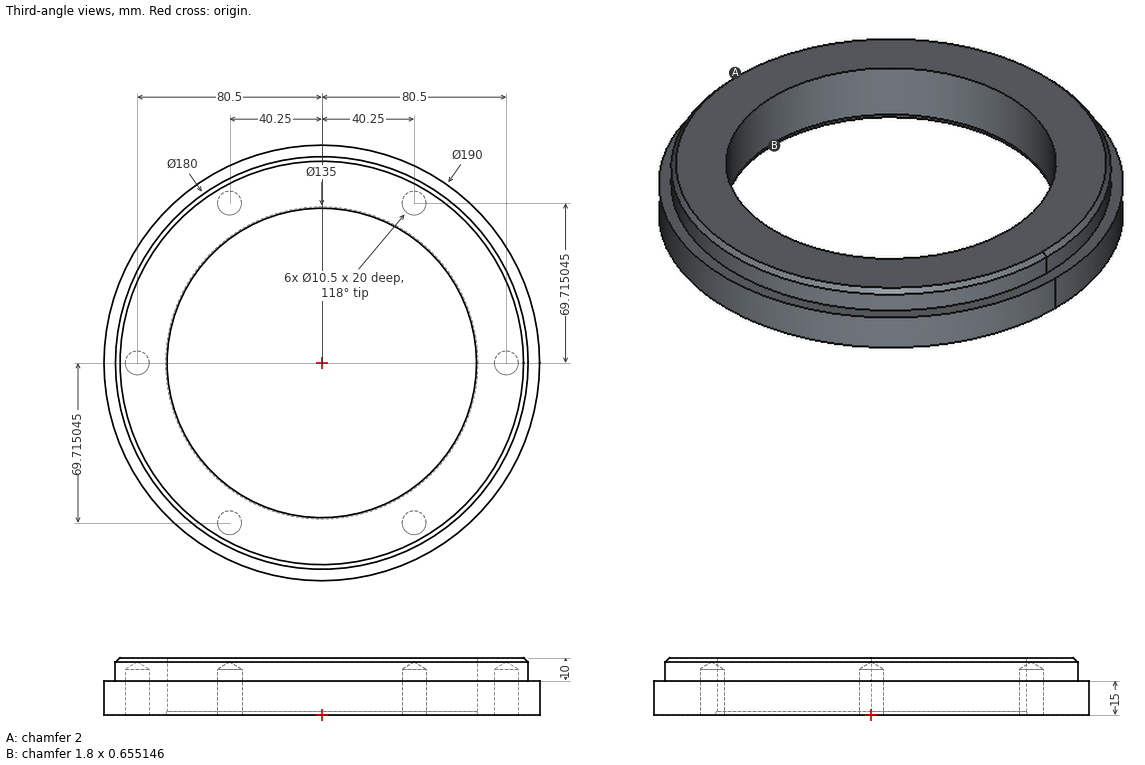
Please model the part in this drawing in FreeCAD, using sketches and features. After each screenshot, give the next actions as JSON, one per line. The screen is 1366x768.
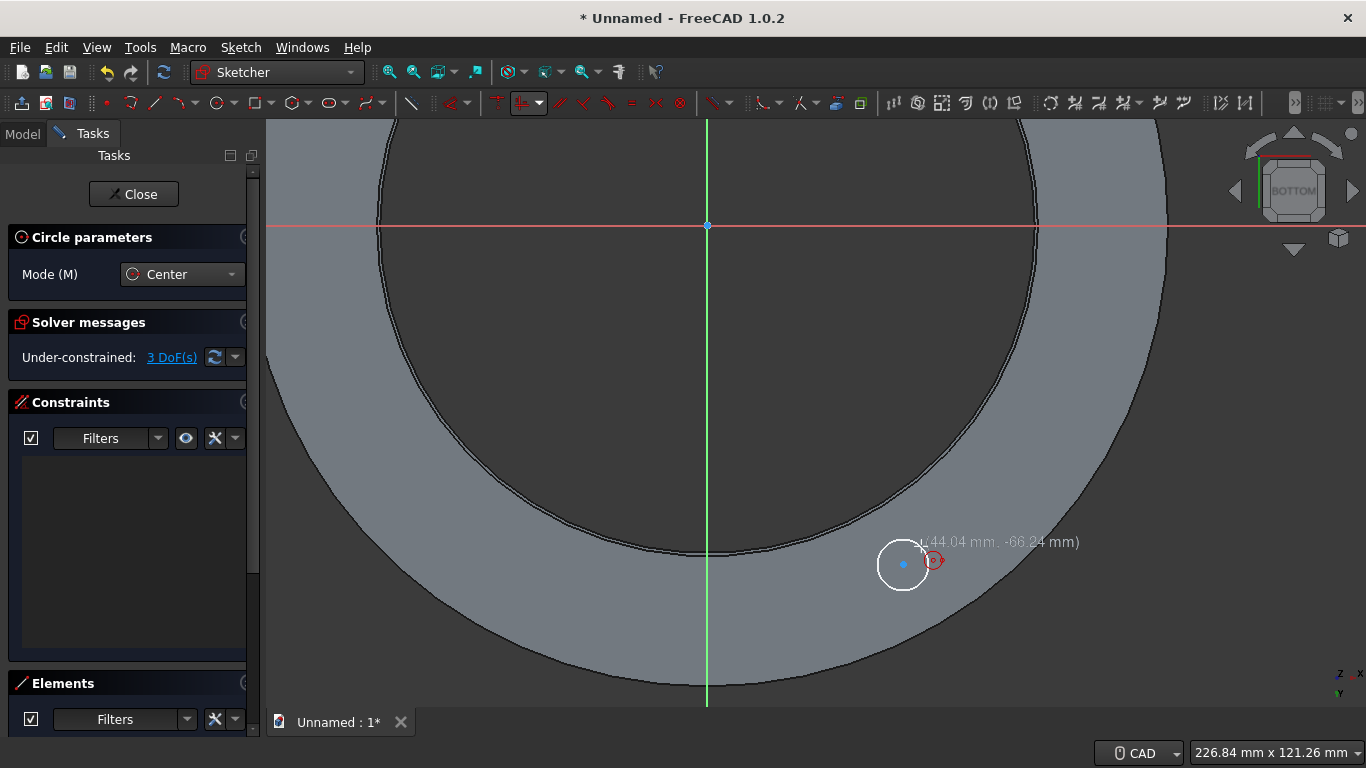
{"action": "left_click", "coordinate": [512, 564]}
{"action": "left_click", "coordinate": [530, 546]}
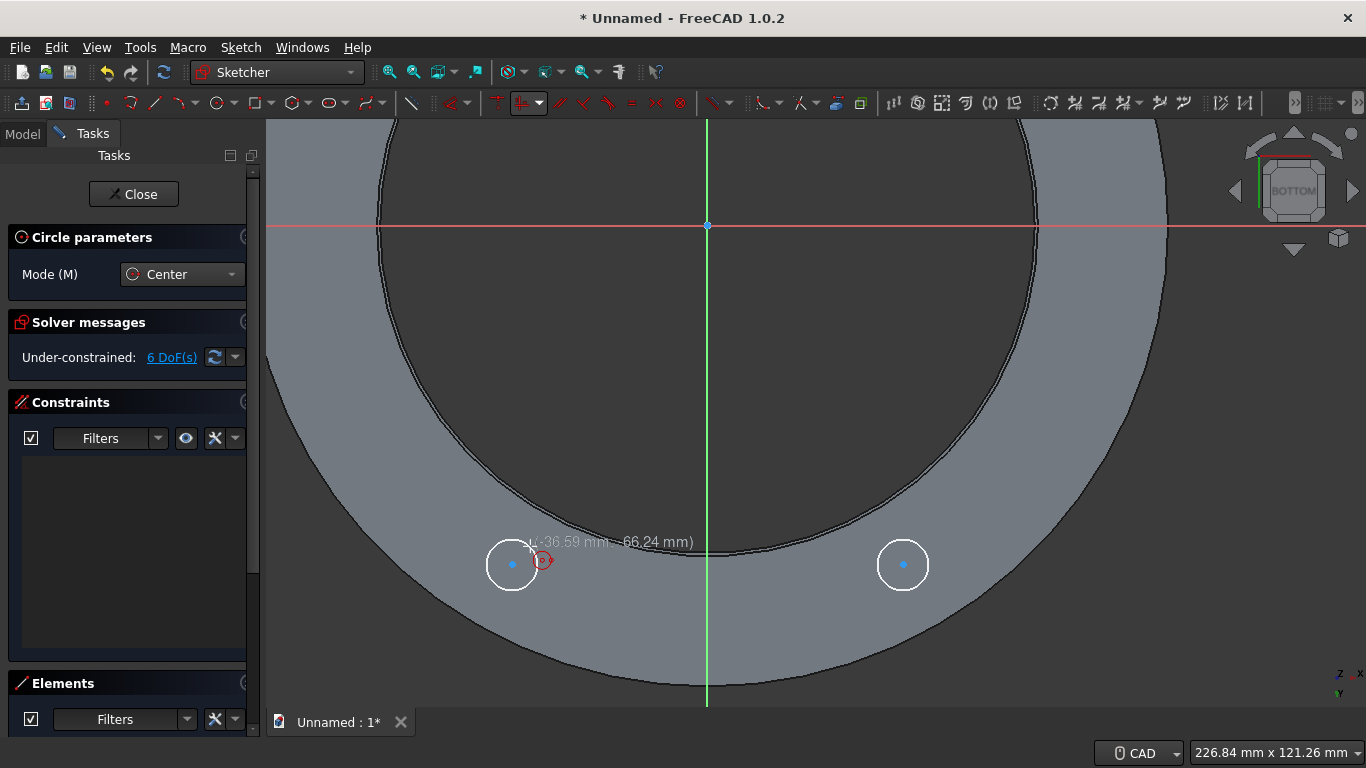
{"action": "left_click", "coordinate": [317, 226]}
{"action": "left_click", "coordinate": [335, 208]}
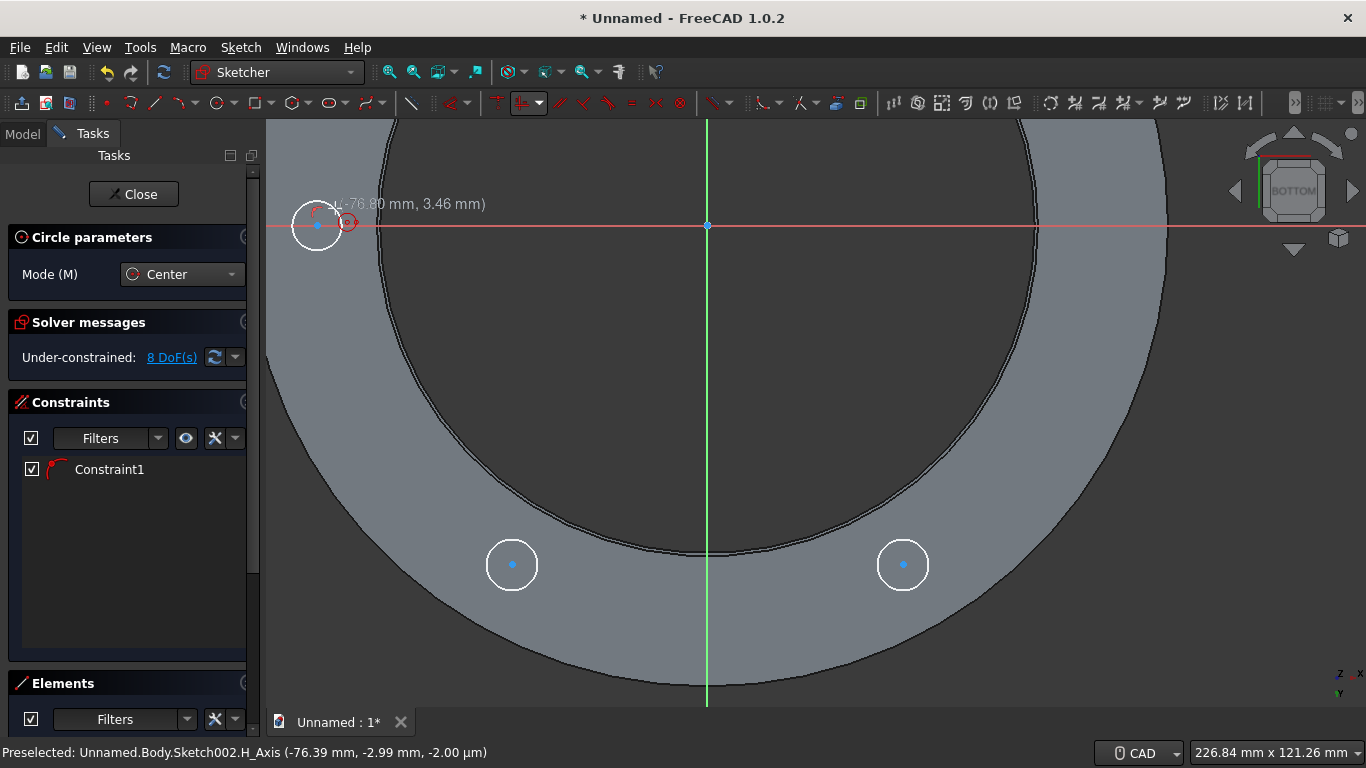
{"action": "scroll", "coordinate": [796, 641], "scroll_direction": "down", "scroll_amount": 3}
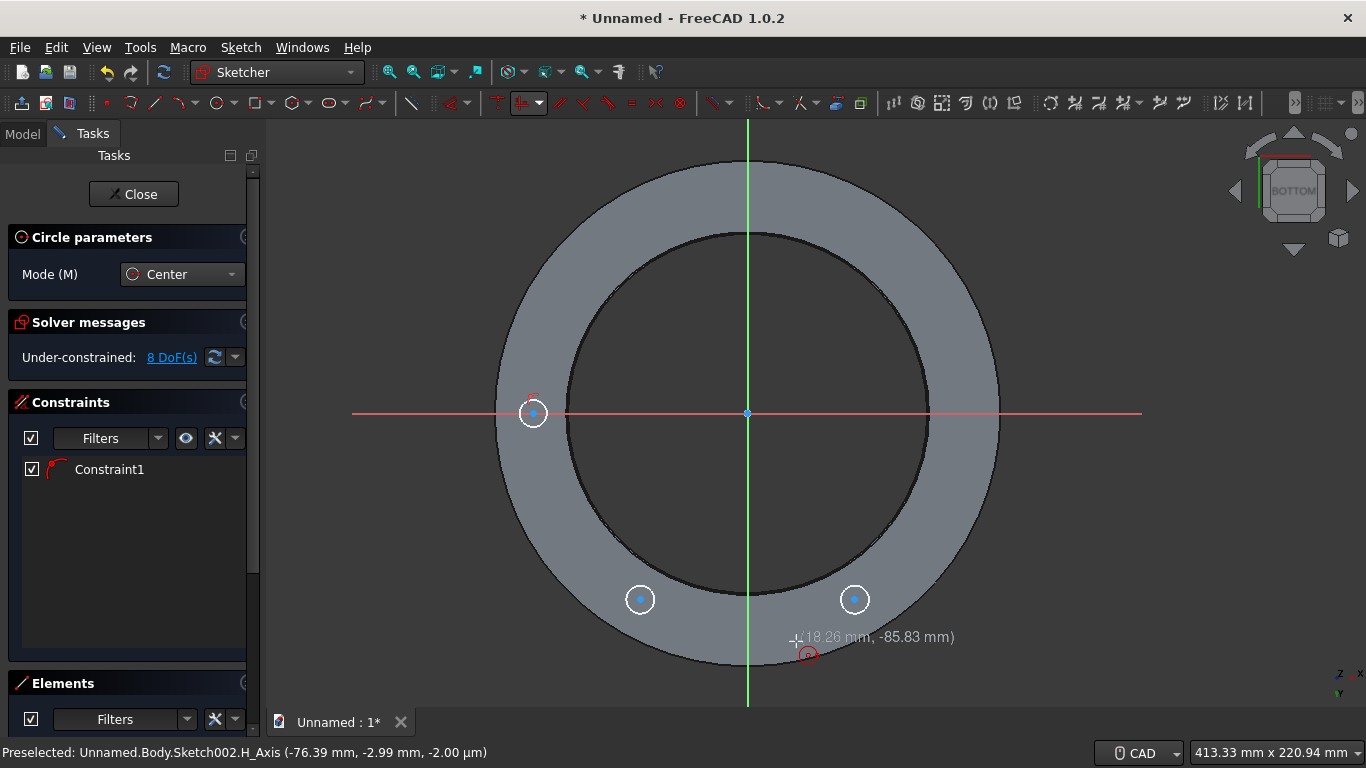
{"action": "scroll", "coordinate": [640, 228], "scroll_direction": "up", "scroll_amount": 3}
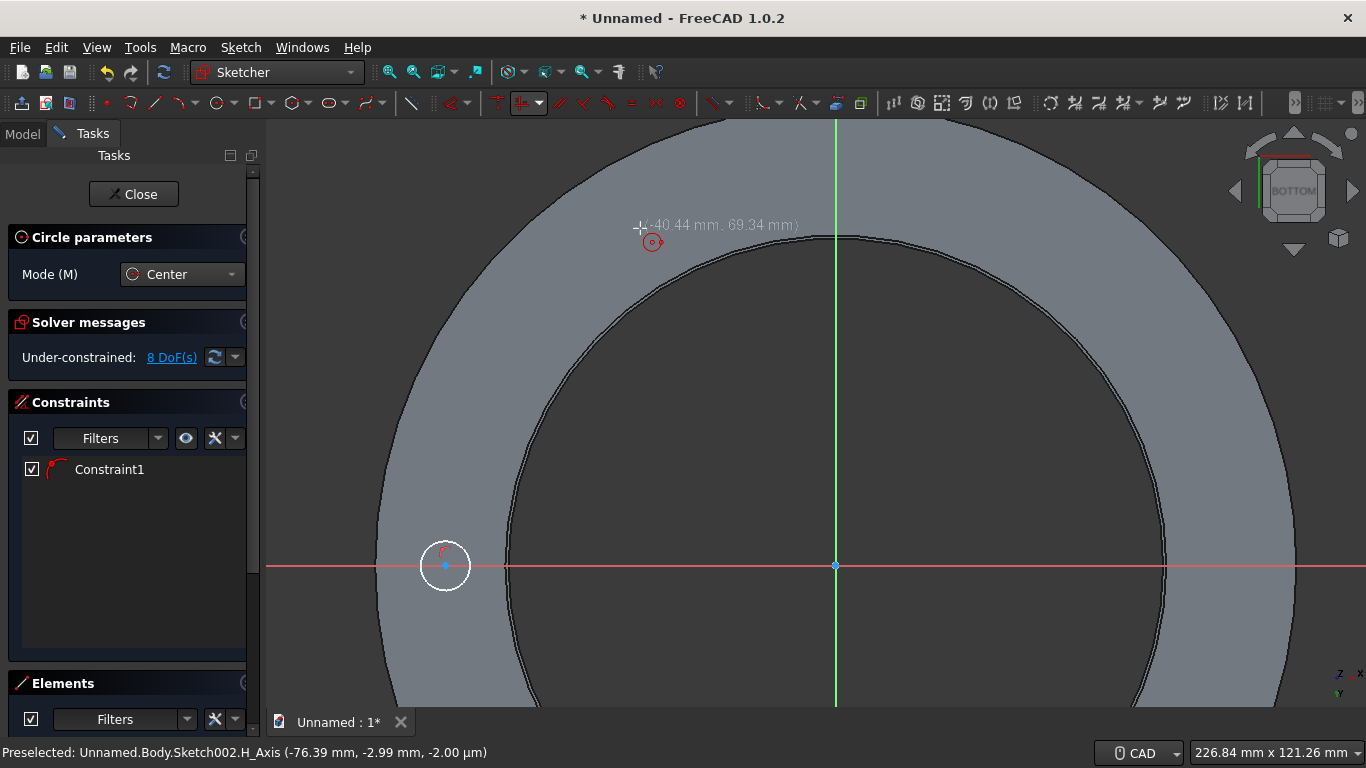
{"action": "left_click", "coordinate": [641, 228]}
{"action": "left_click", "coordinate": [659, 210]}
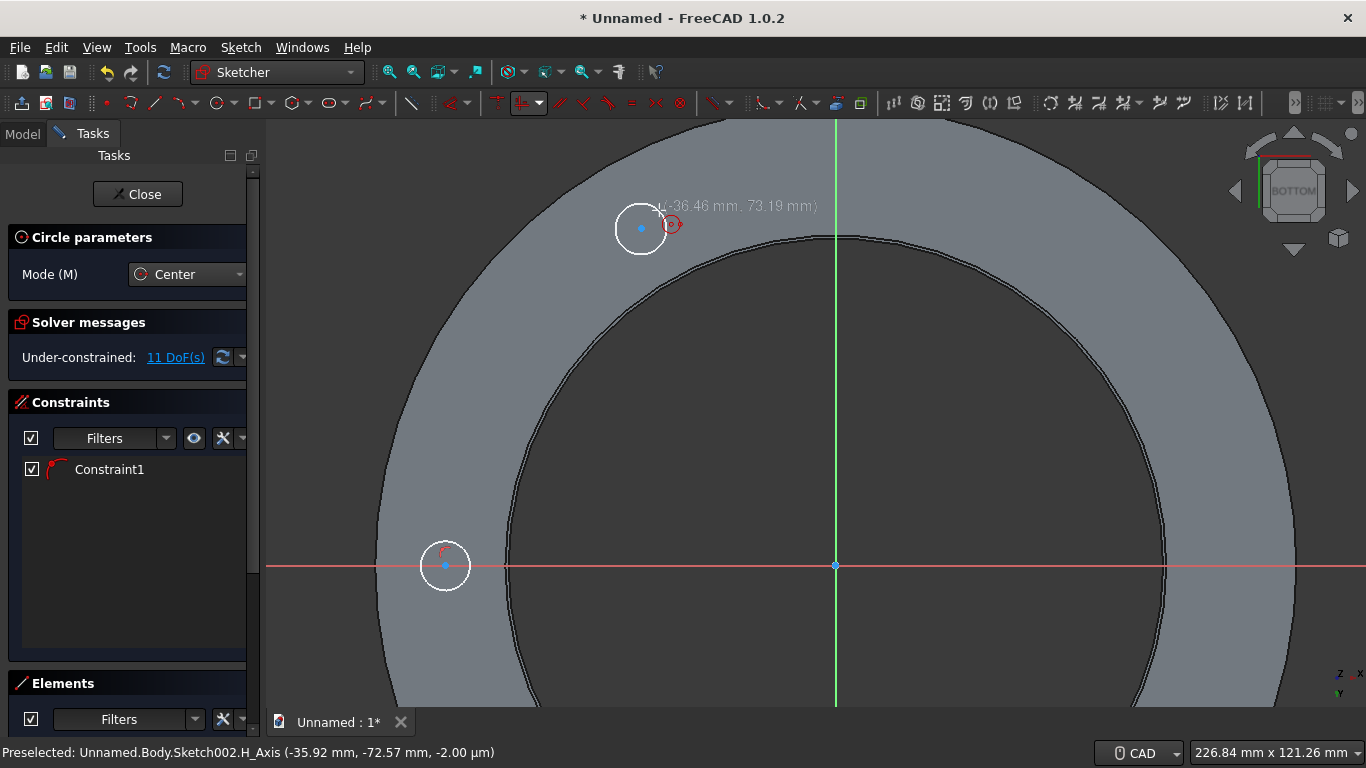
{"action": "scroll", "coordinate": [640, 227], "scroll_direction": "down", "scroll_amount": 3}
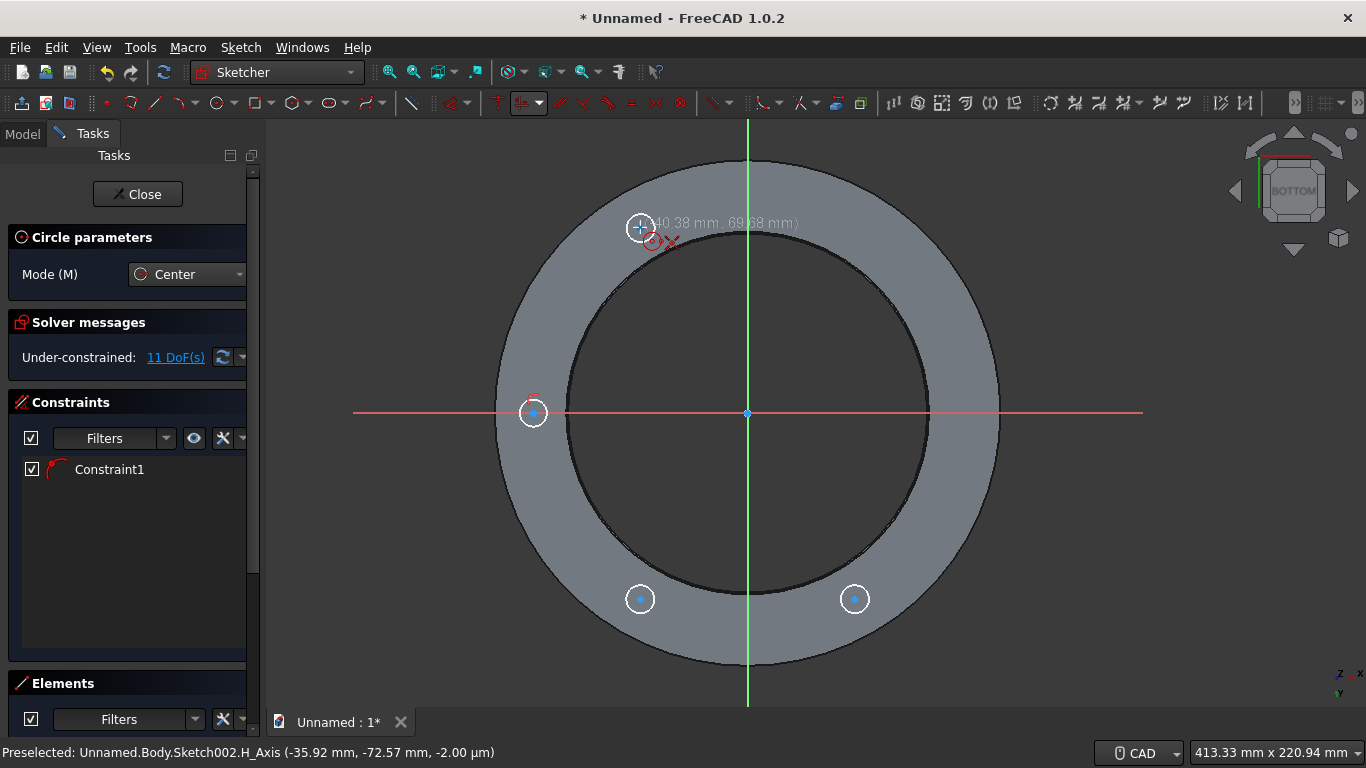
{"action": "scroll", "coordinate": [962, 413], "scroll_direction": "up", "scroll_amount": 3}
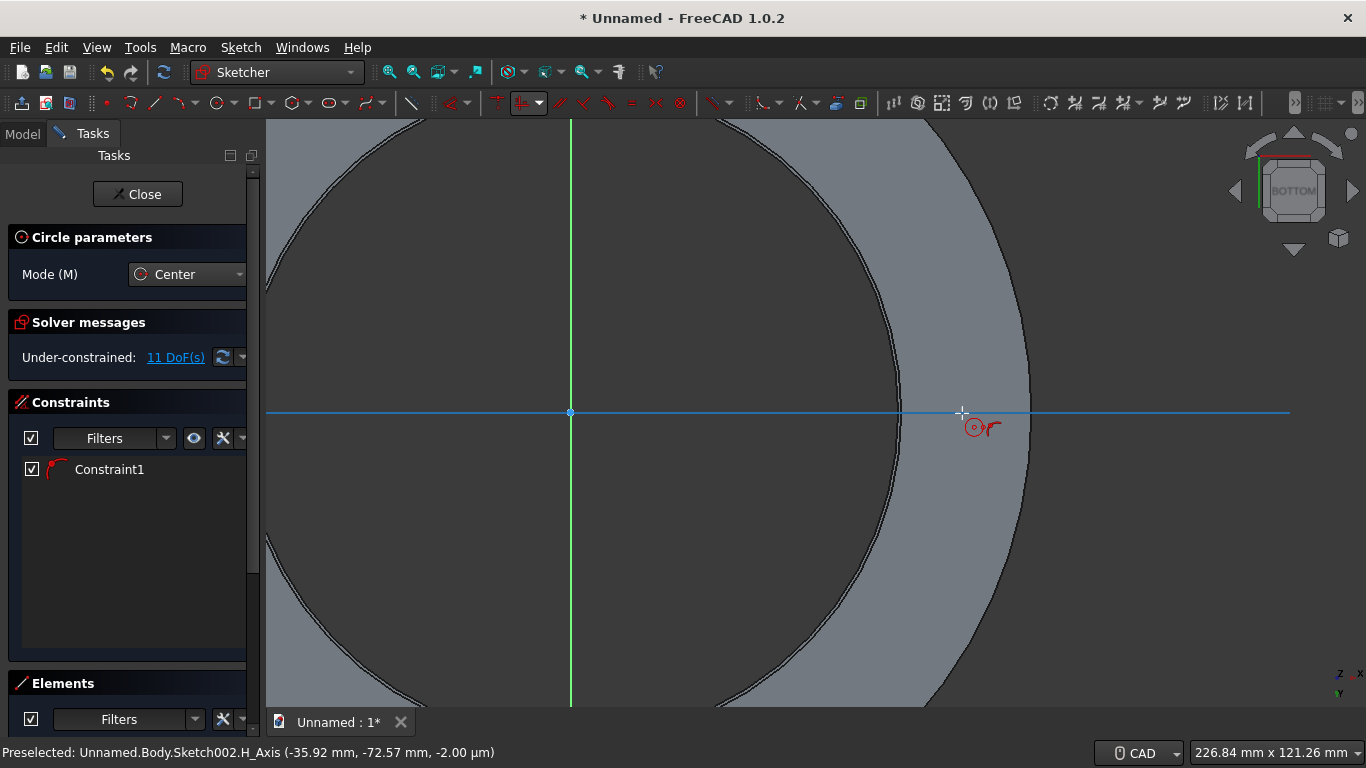
{"action": "left_click", "coordinate": [961, 413]}
{"action": "left_click", "coordinate": [979, 395]}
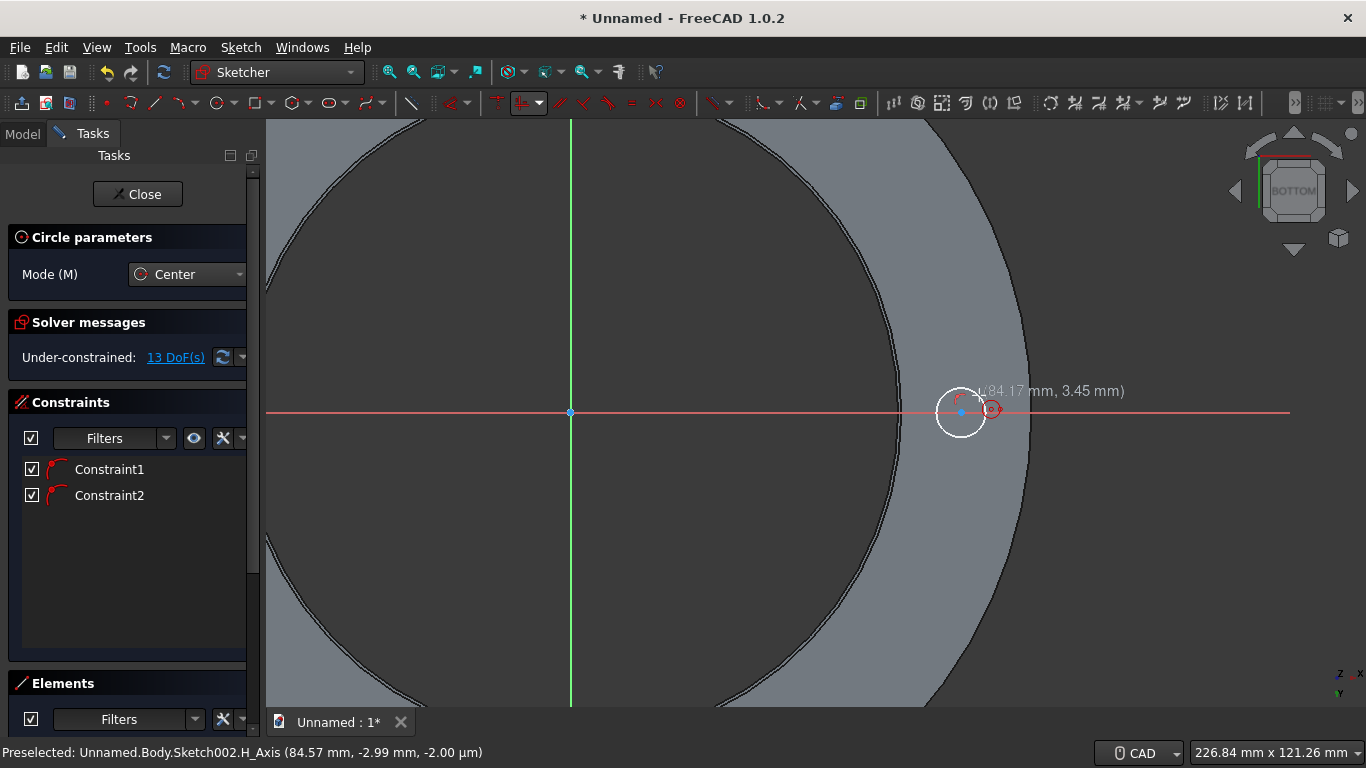
{"action": "scroll", "coordinate": [962, 413], "scroll_direction": "down", "scroll_amount": 3}